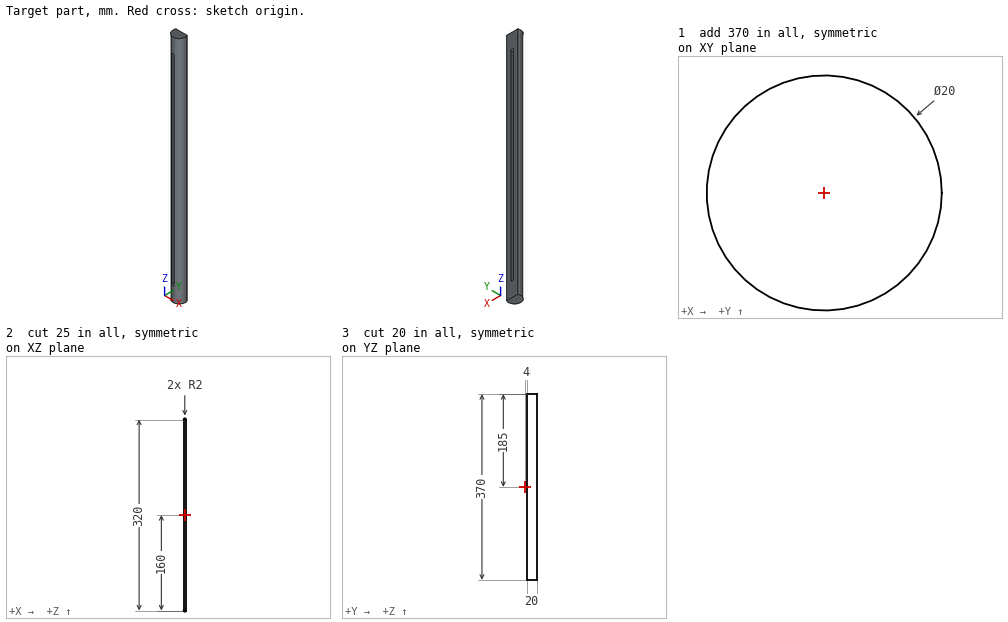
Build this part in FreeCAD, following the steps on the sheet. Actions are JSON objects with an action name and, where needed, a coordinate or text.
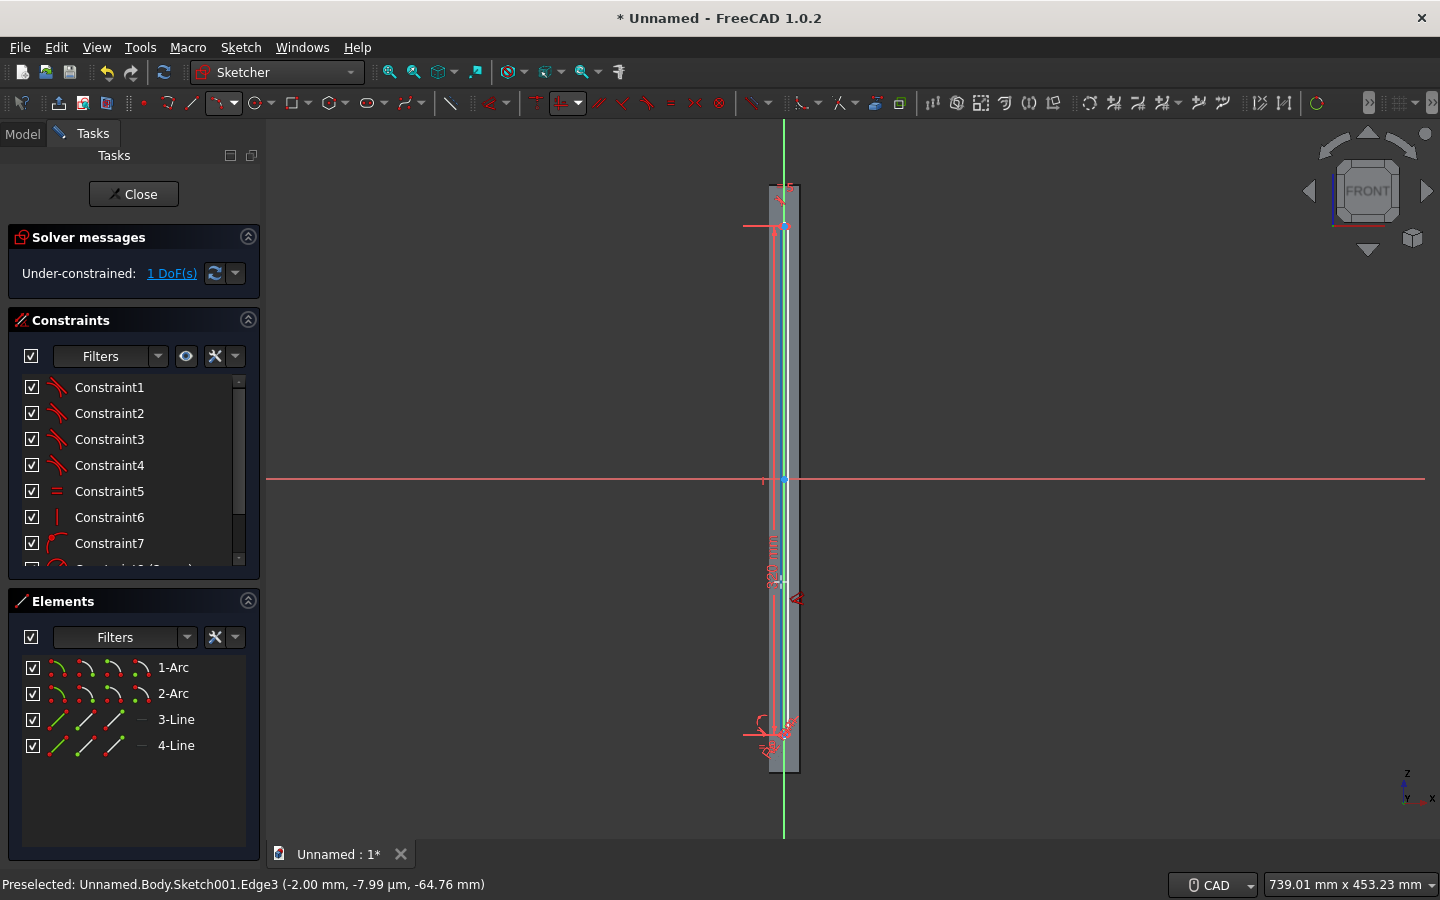
{"action": "scroll", "coordinate": [781, 735], "scroll_direction": "up", "scroll_amount": 7}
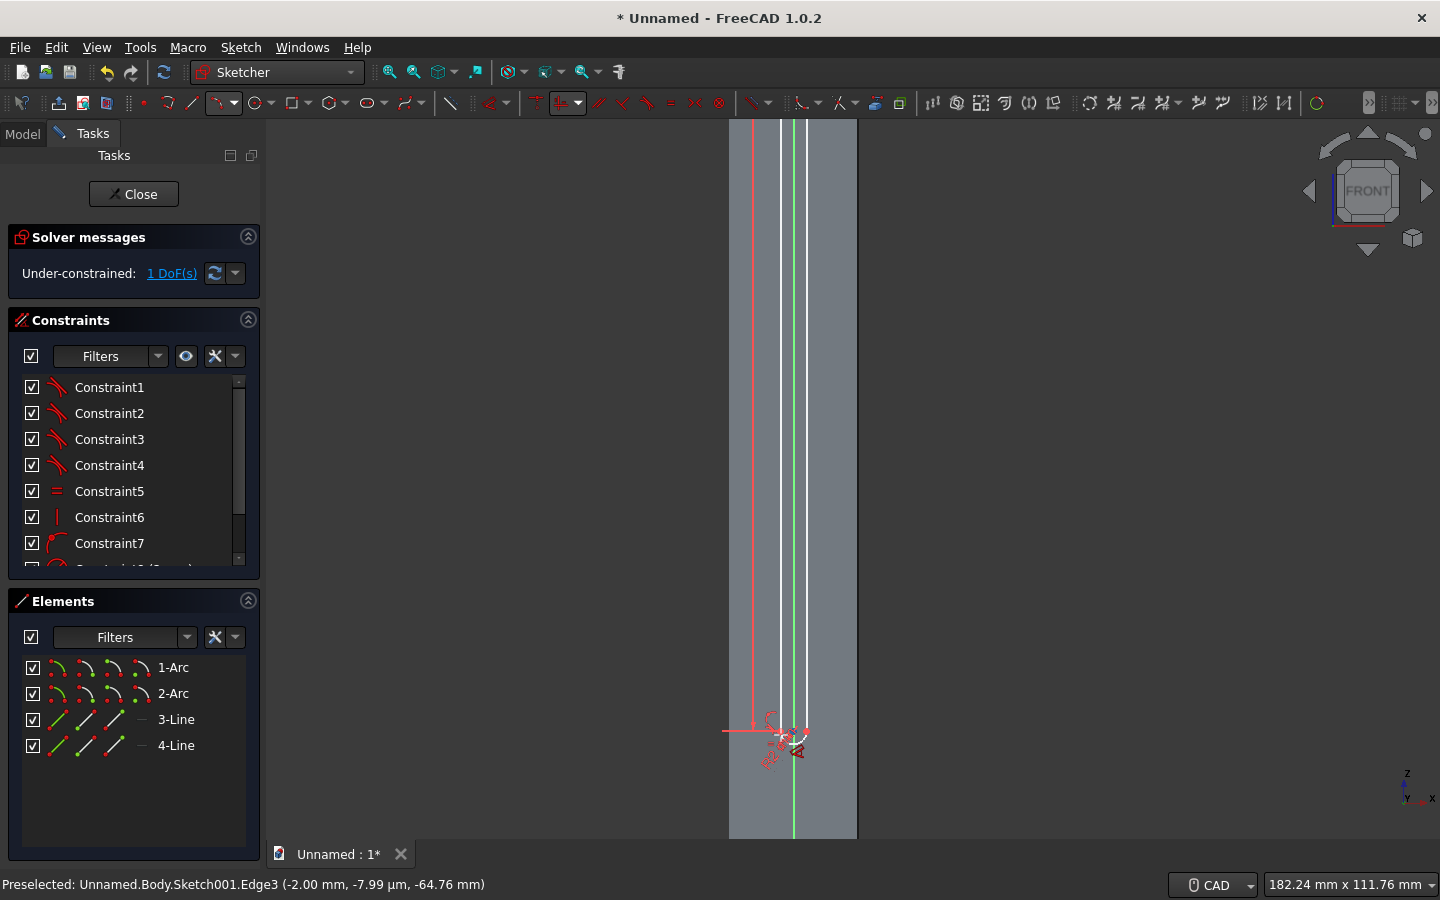
{"action": "left_click", "coordinate": [781, 731]}
{"action": "left_click", "coordinate": [747, 439]}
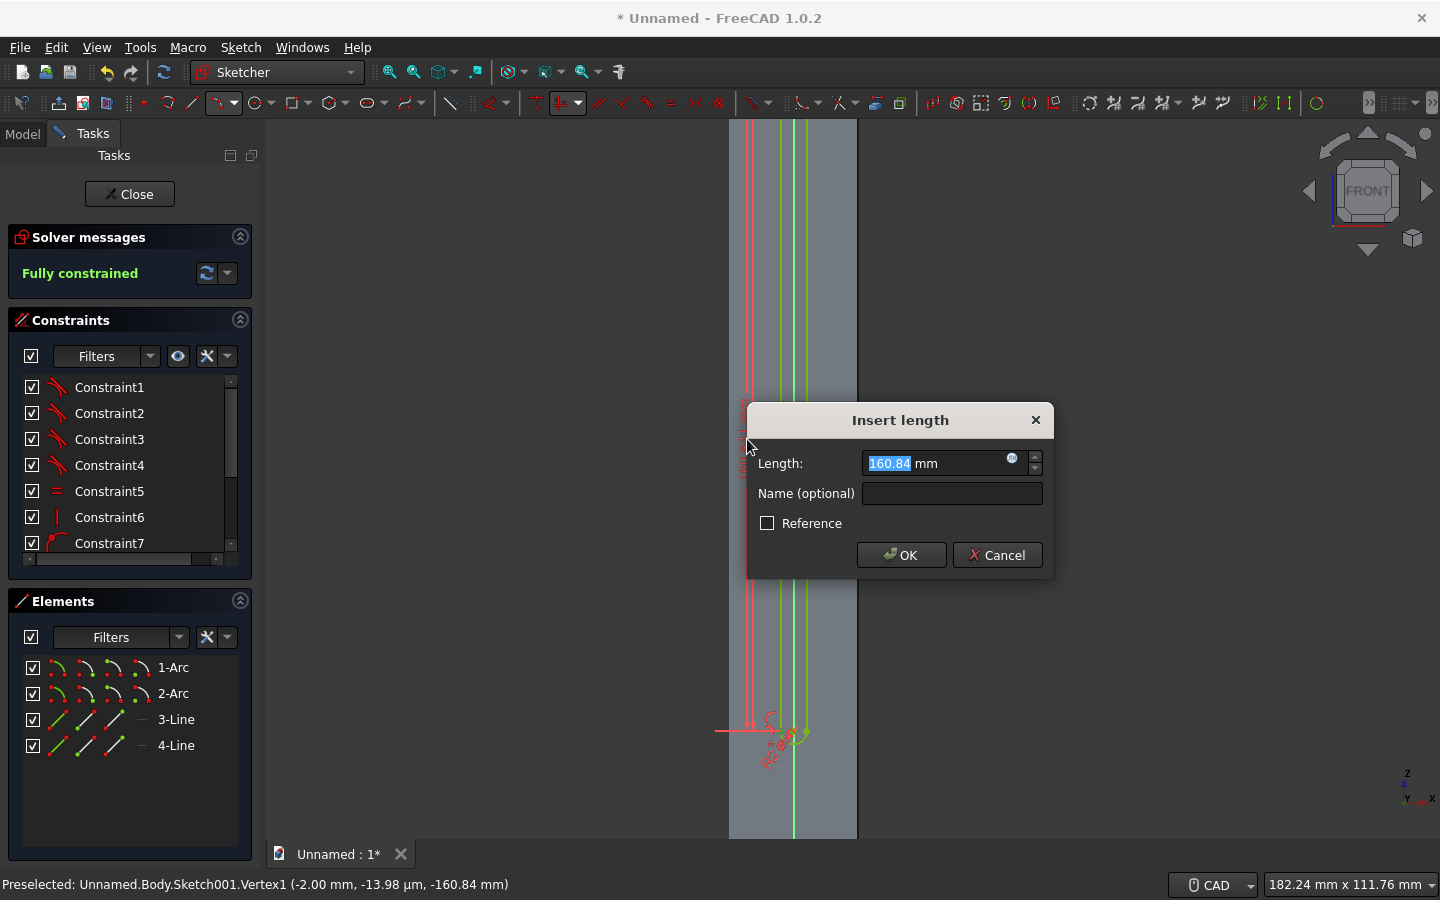
{"action": "type", "text": "160"}
{"action": "key", "text": "Return"}
{"action": "key", "text": "Escape"}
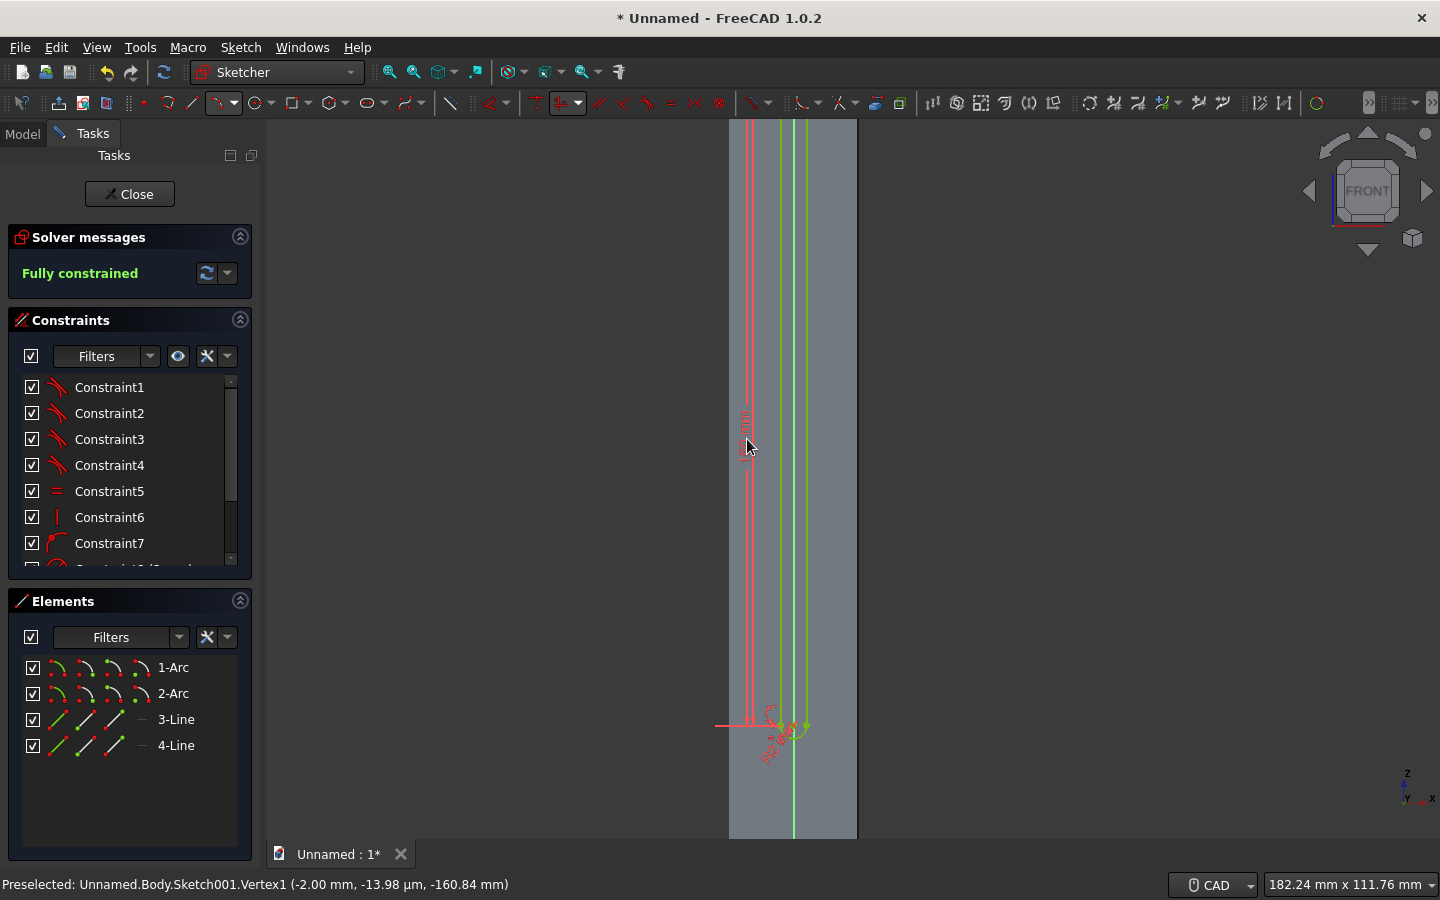
{"action": "left_click", "coordinate": [130, 194]}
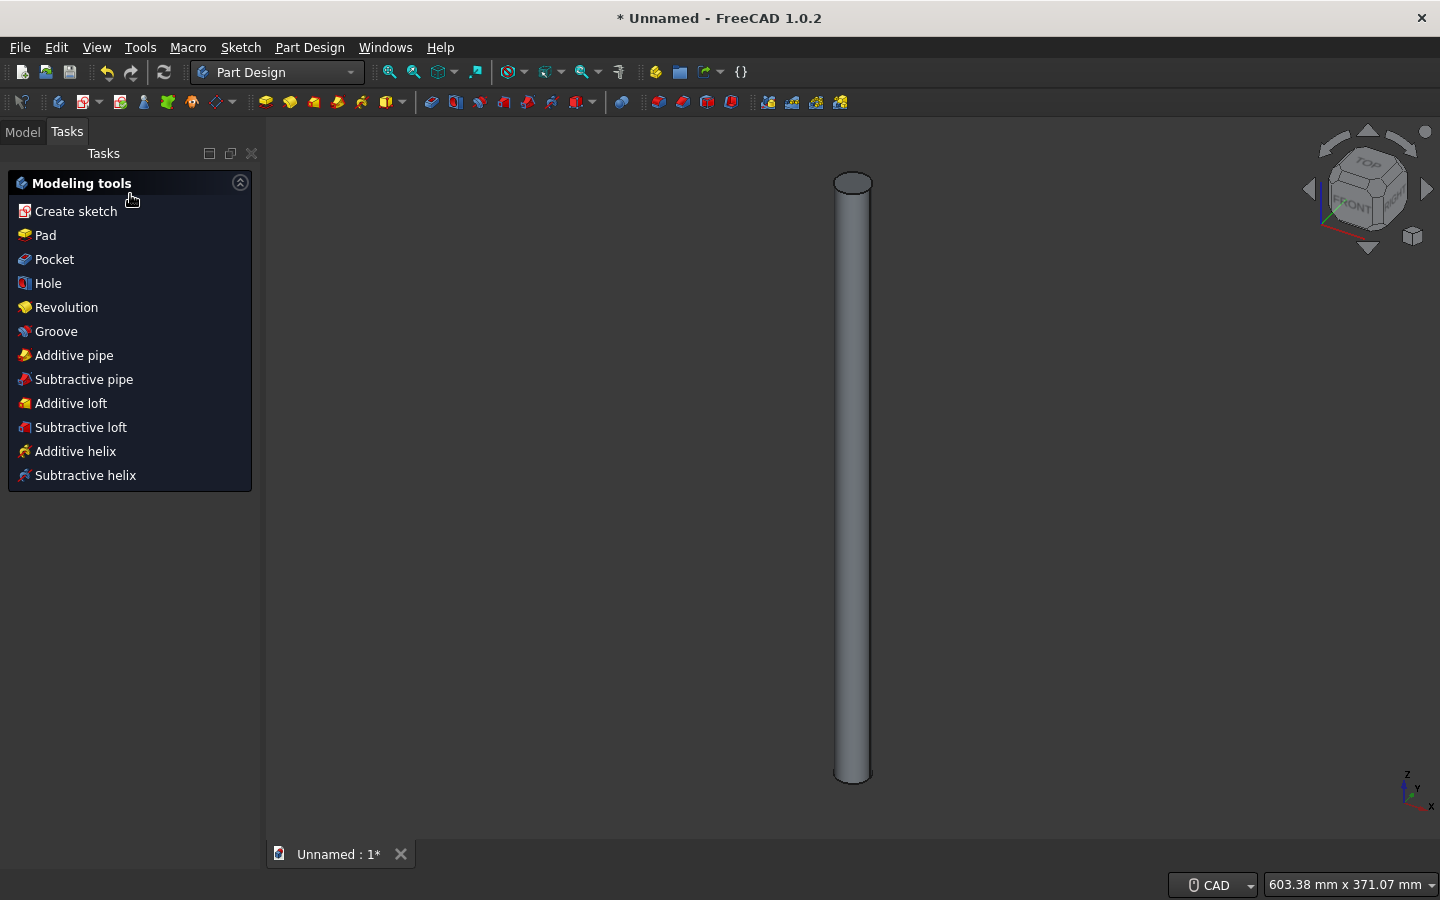
{"action": "left_click", "coordinate": [432, 102]}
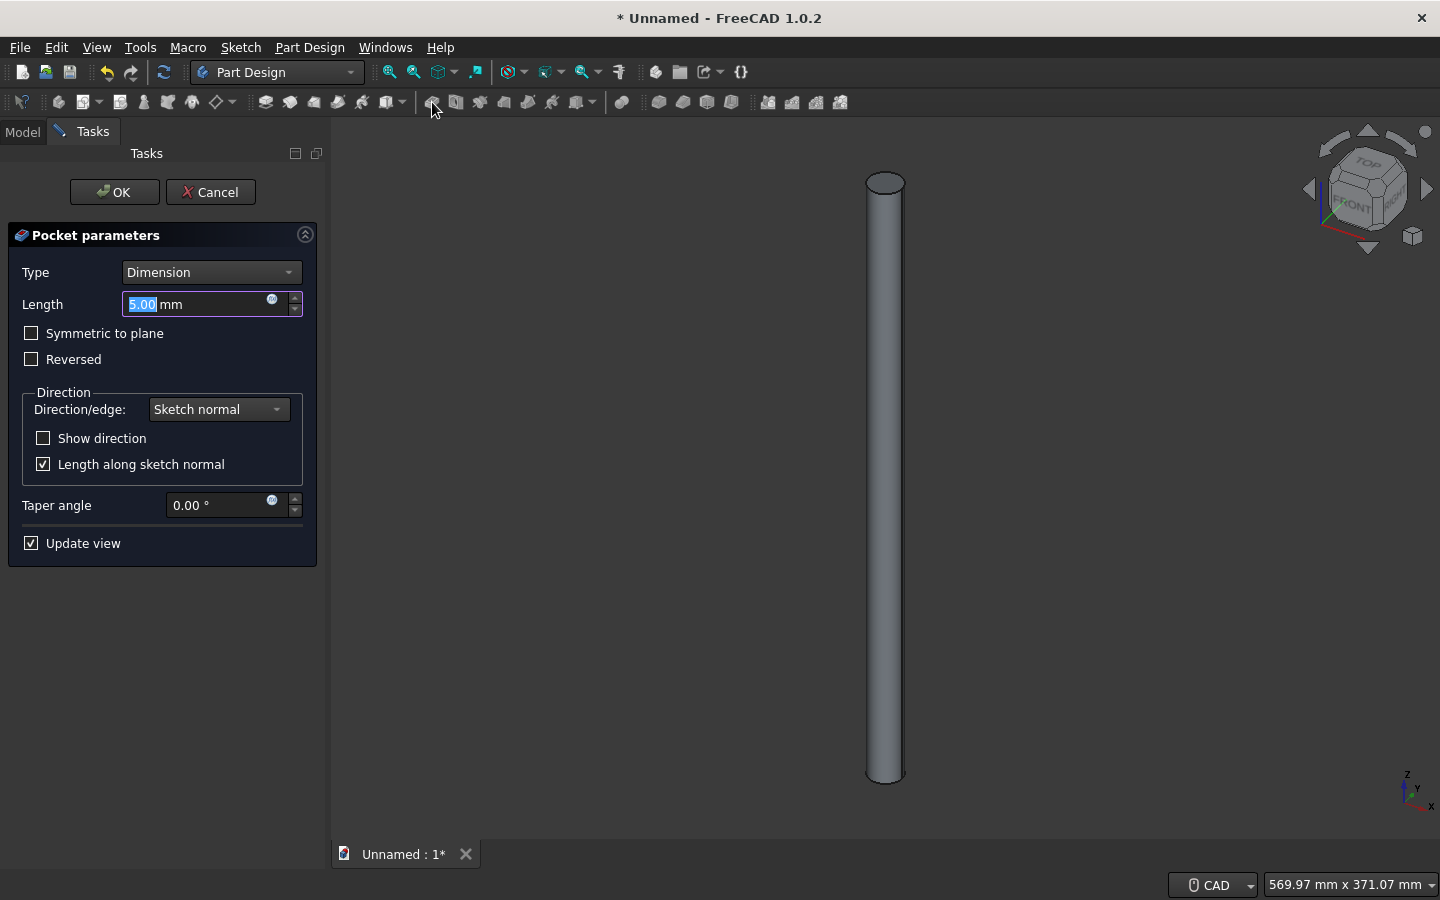
{"action": "type", "text": "25"}
{"action": "key", "text": "Tab"}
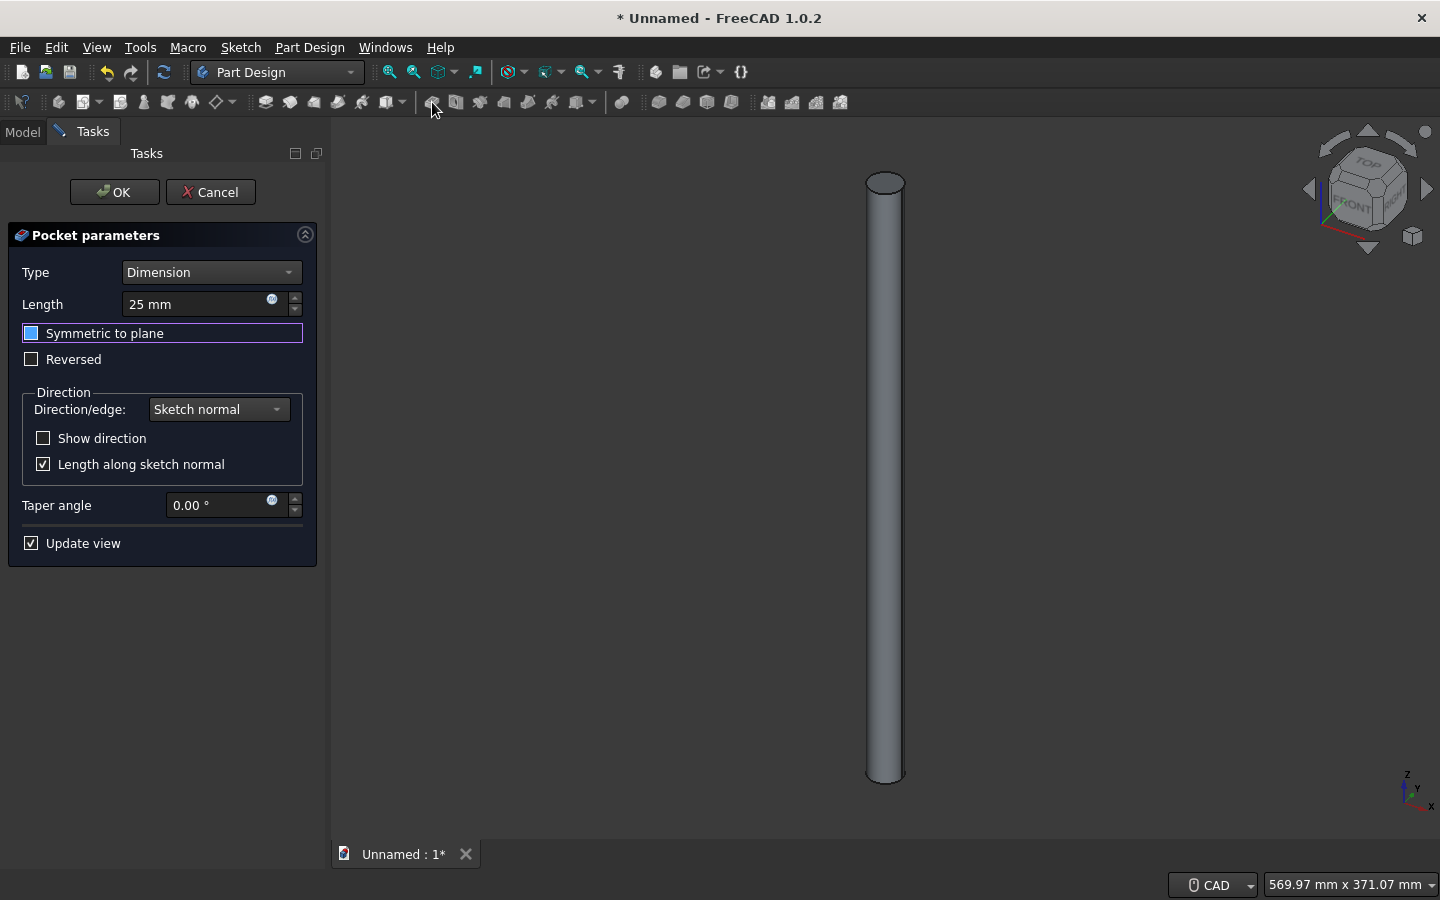
{"action": "left_click", "coordinate": [30, 333]}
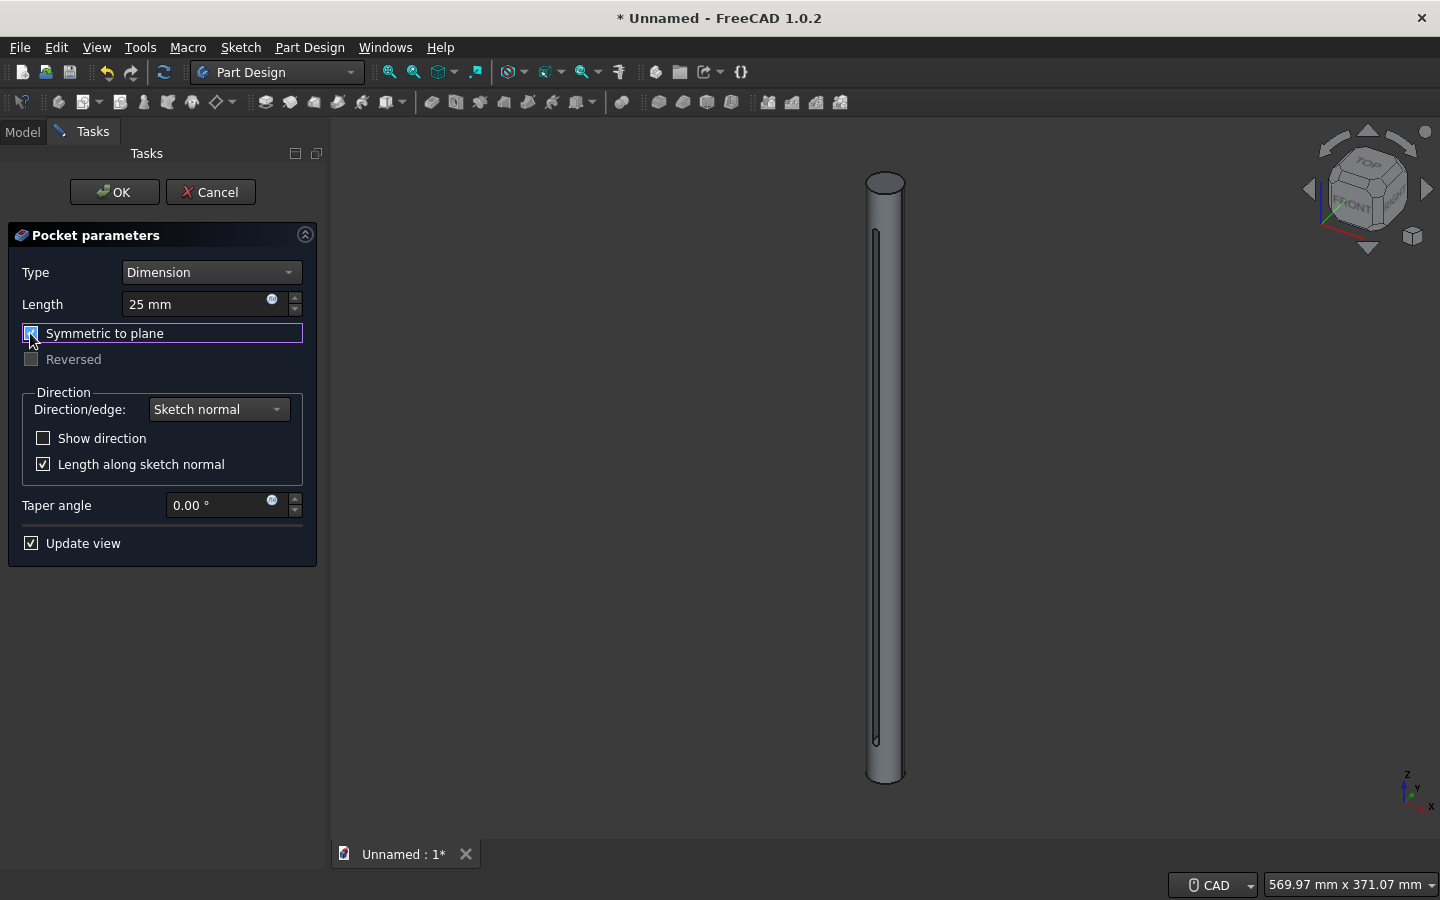
{"action": "left_click", "coordinate": [115, 192]}